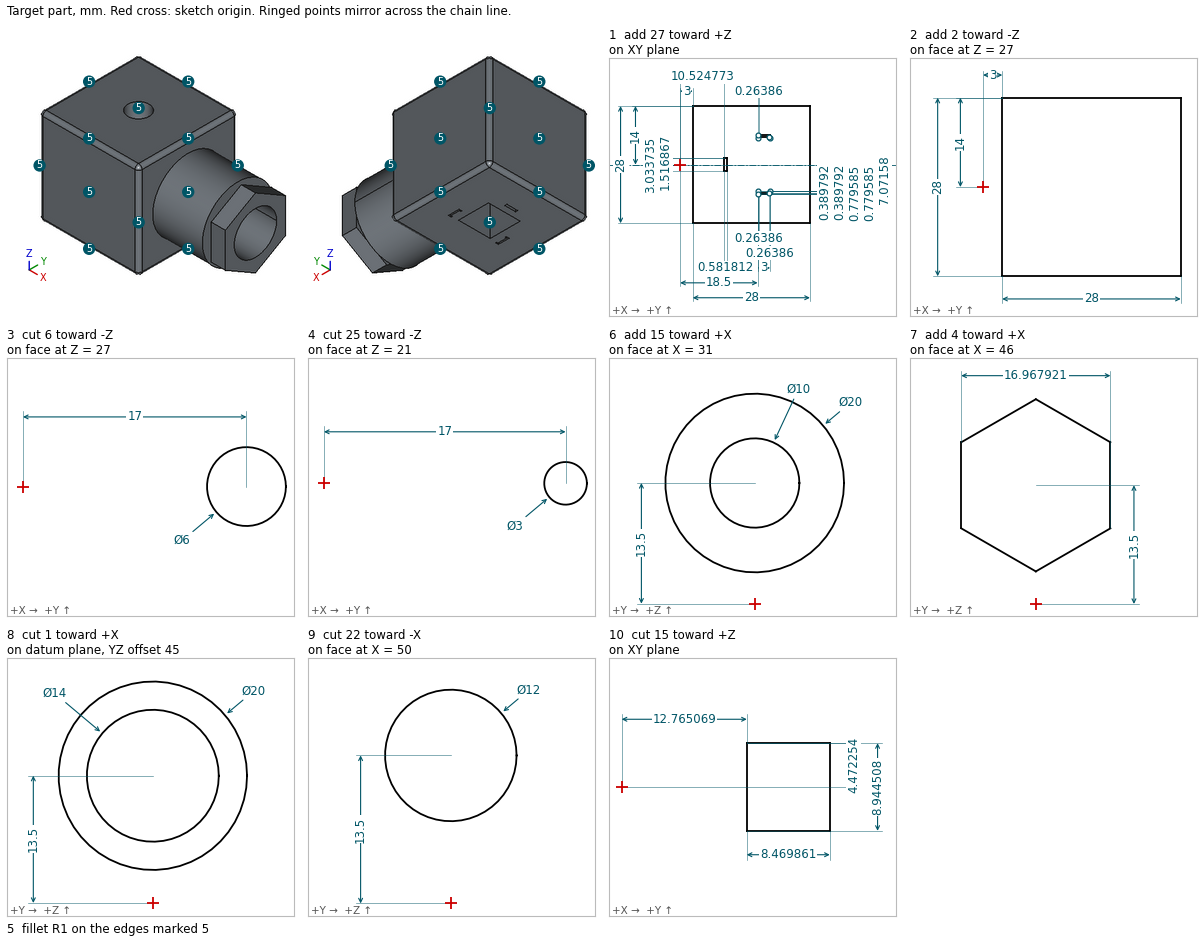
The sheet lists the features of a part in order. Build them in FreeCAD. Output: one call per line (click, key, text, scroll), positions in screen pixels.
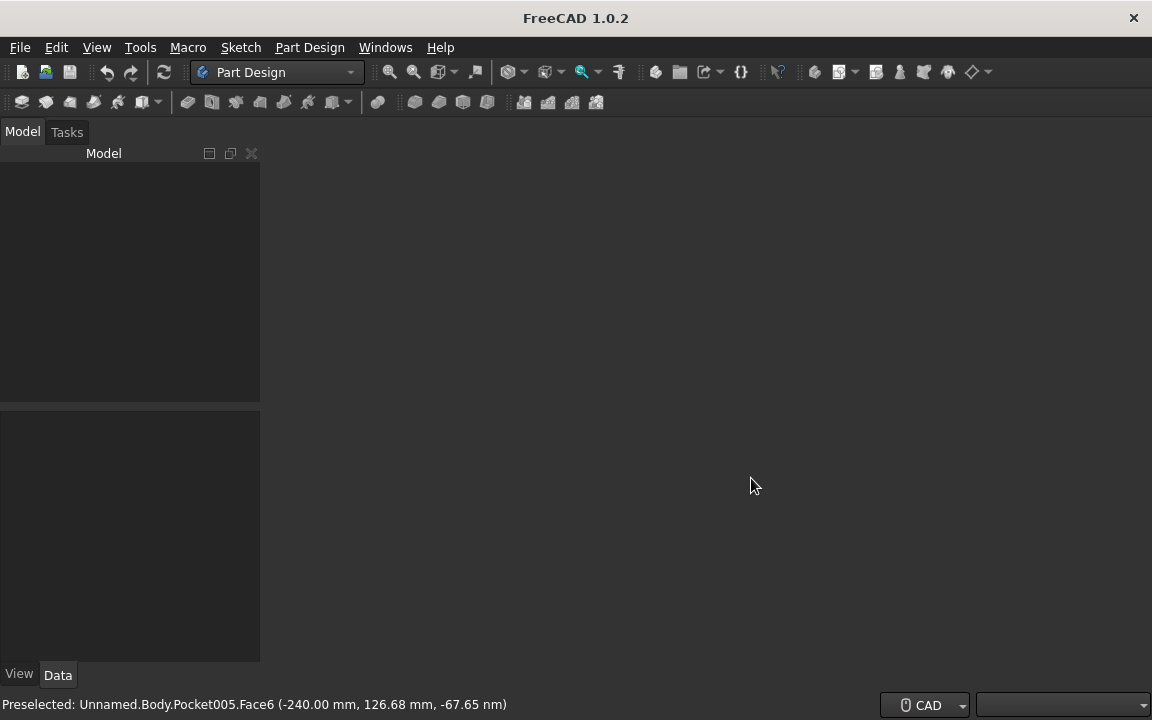
click(22, 72)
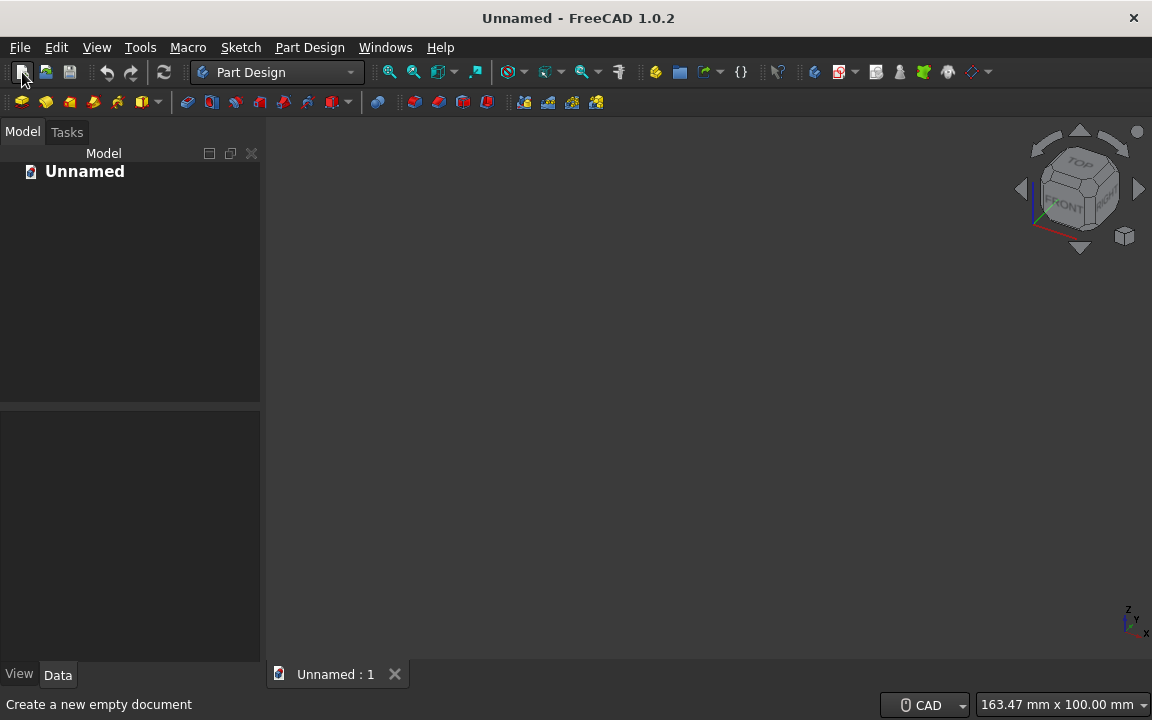
click(840, 72)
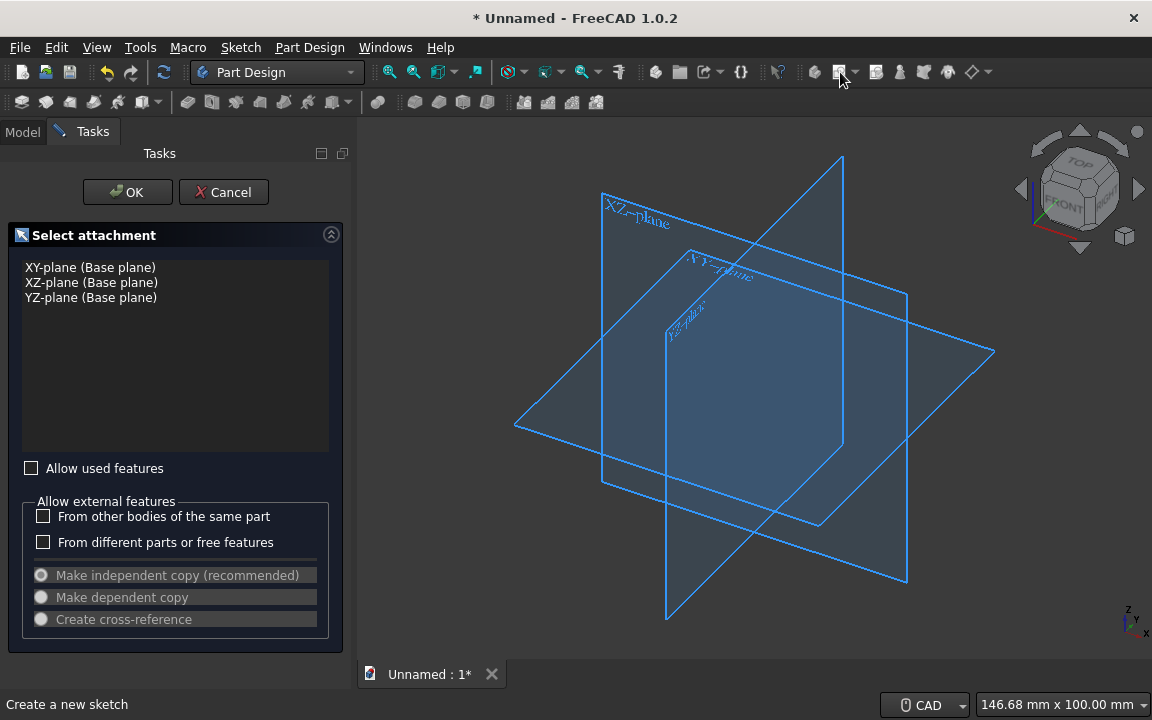
click(82, 268)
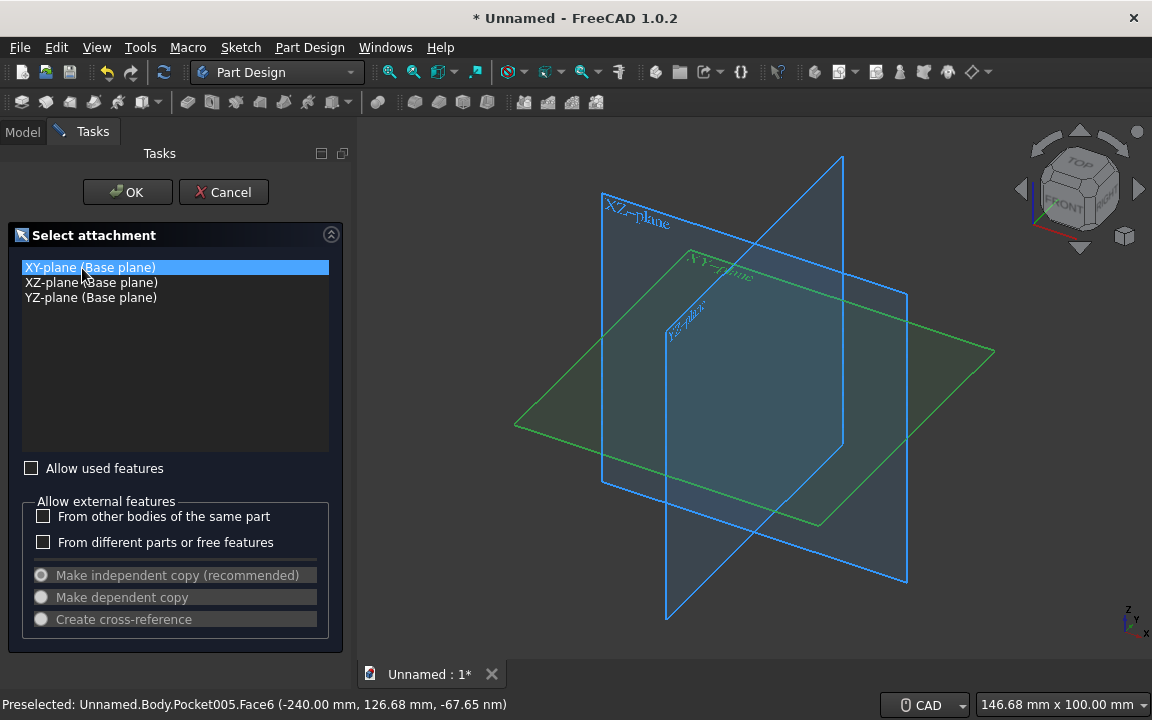
click(128, 192)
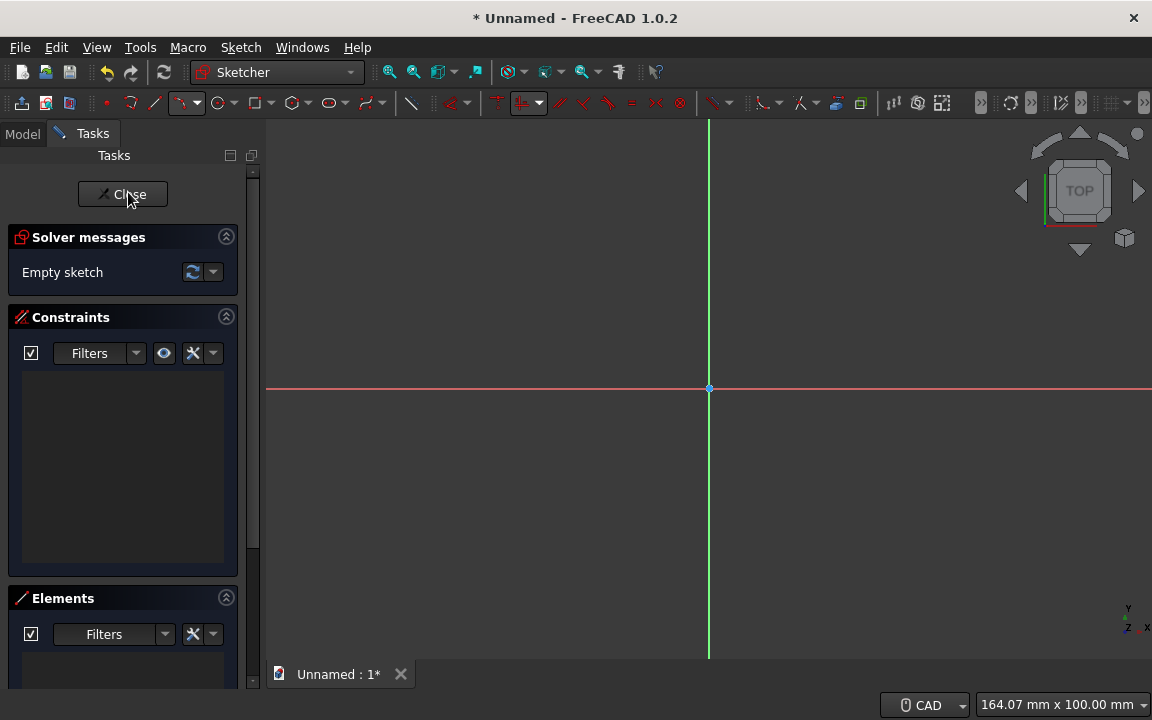
scroll(917, 389, up, 4)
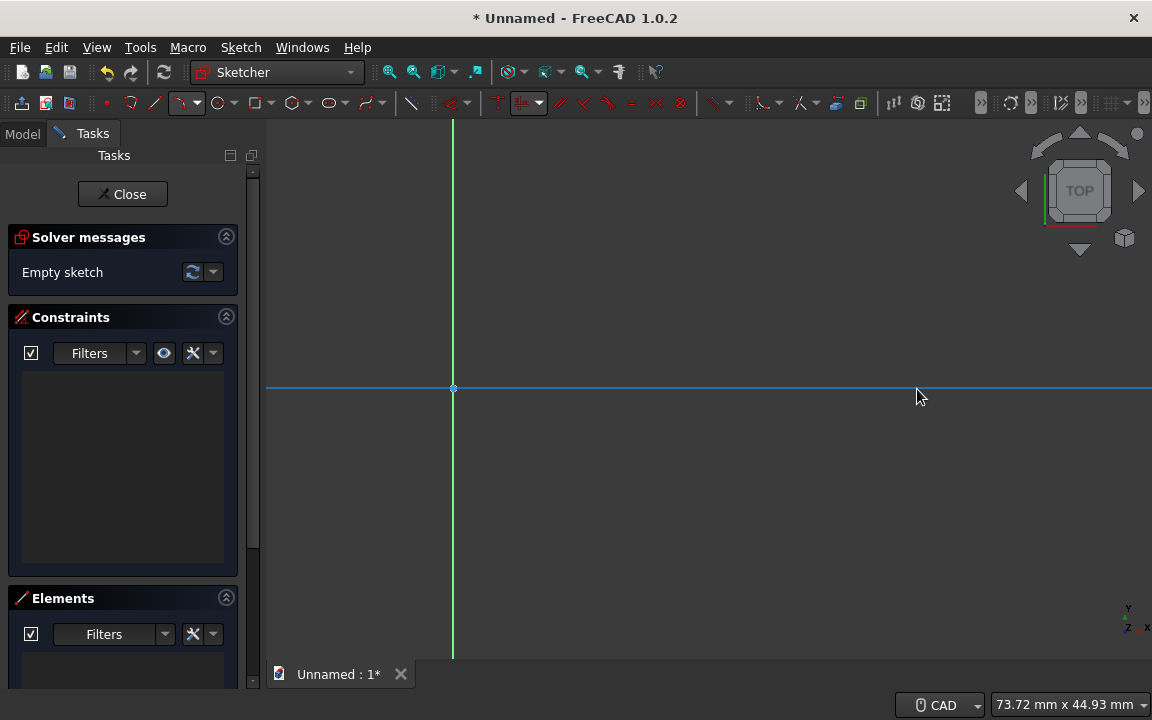
click(256, 104)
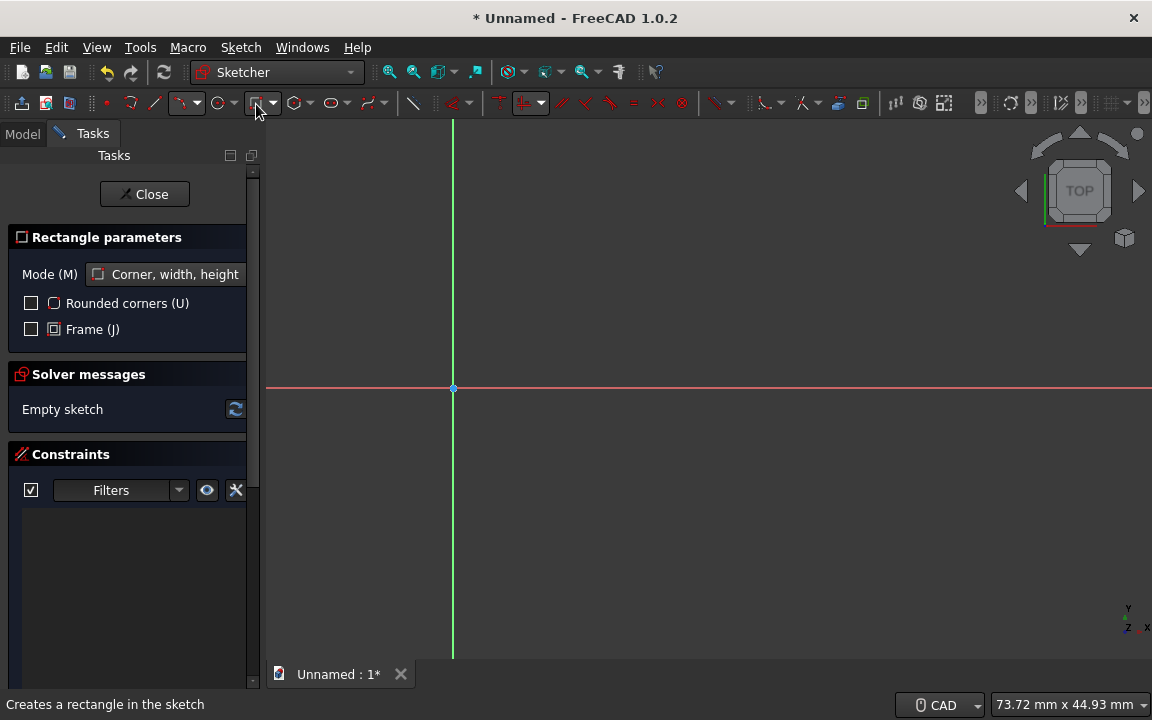
click(489, 220)
click(826, 557)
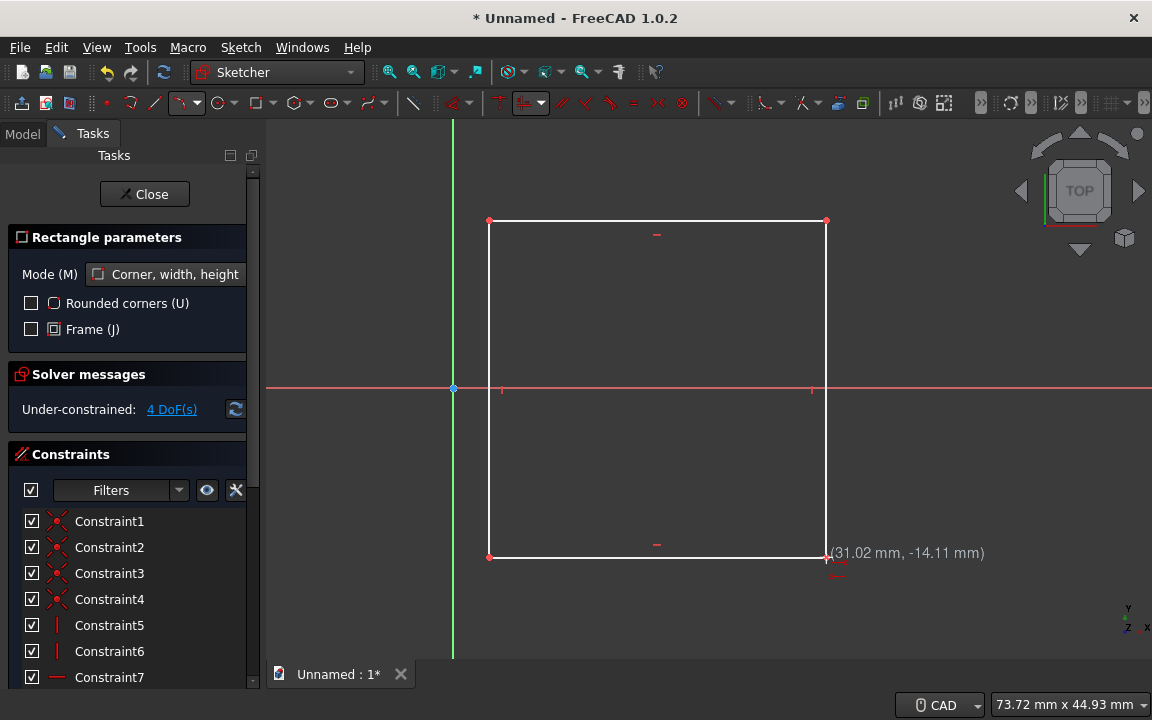
click(132, 104)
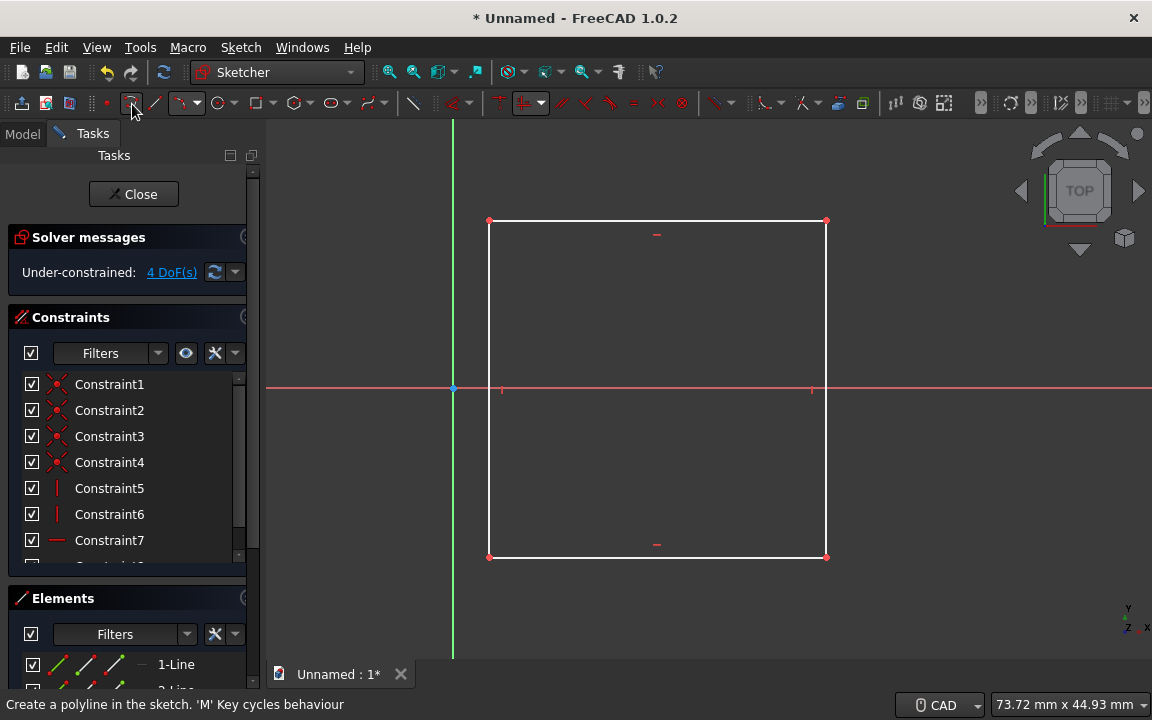
click(676, 464)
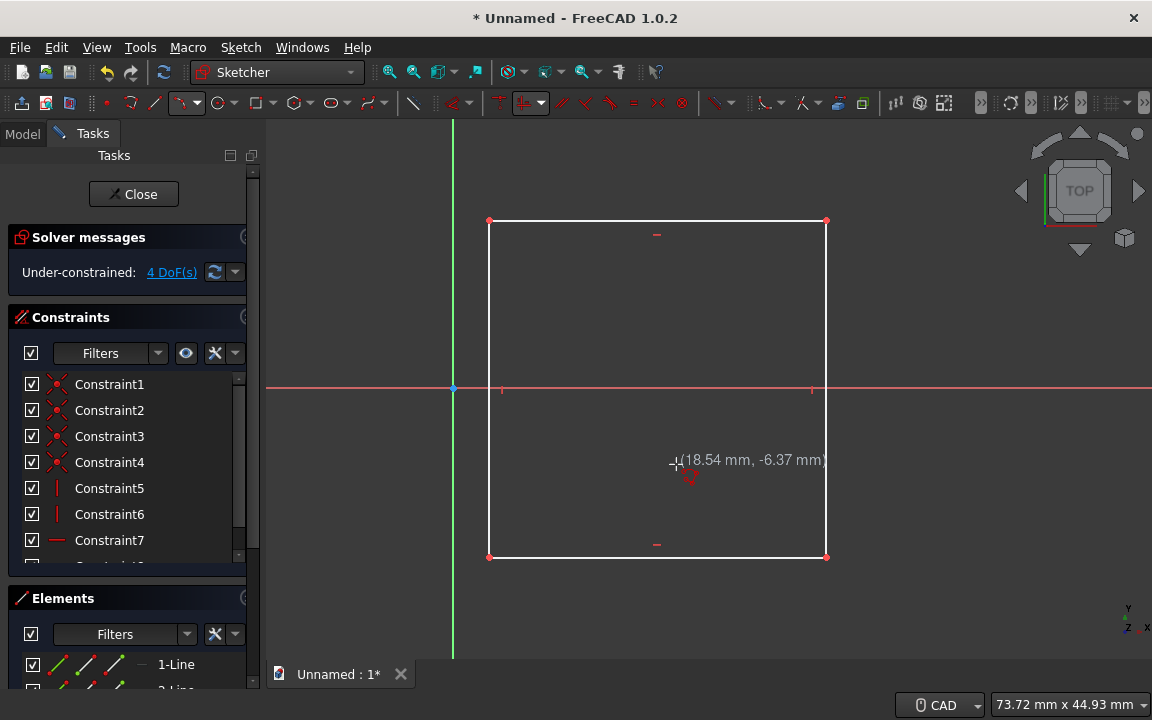
scroll(679, 464, up, 9)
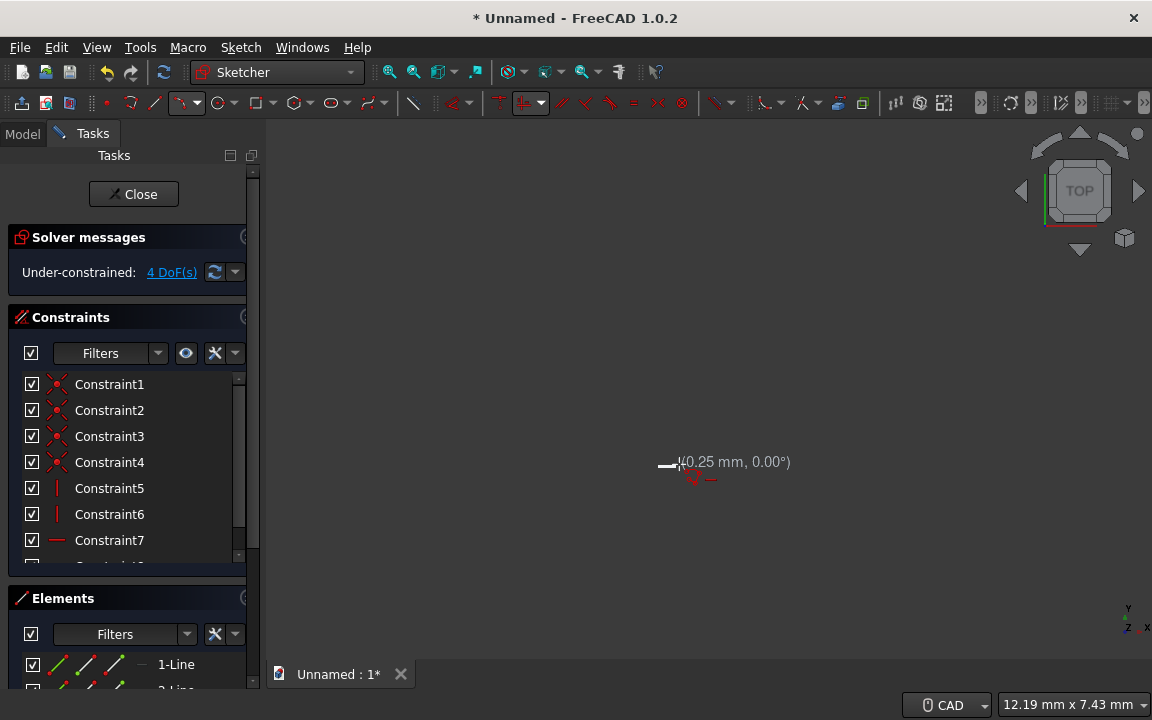
click(675, 461)
click(675, 489)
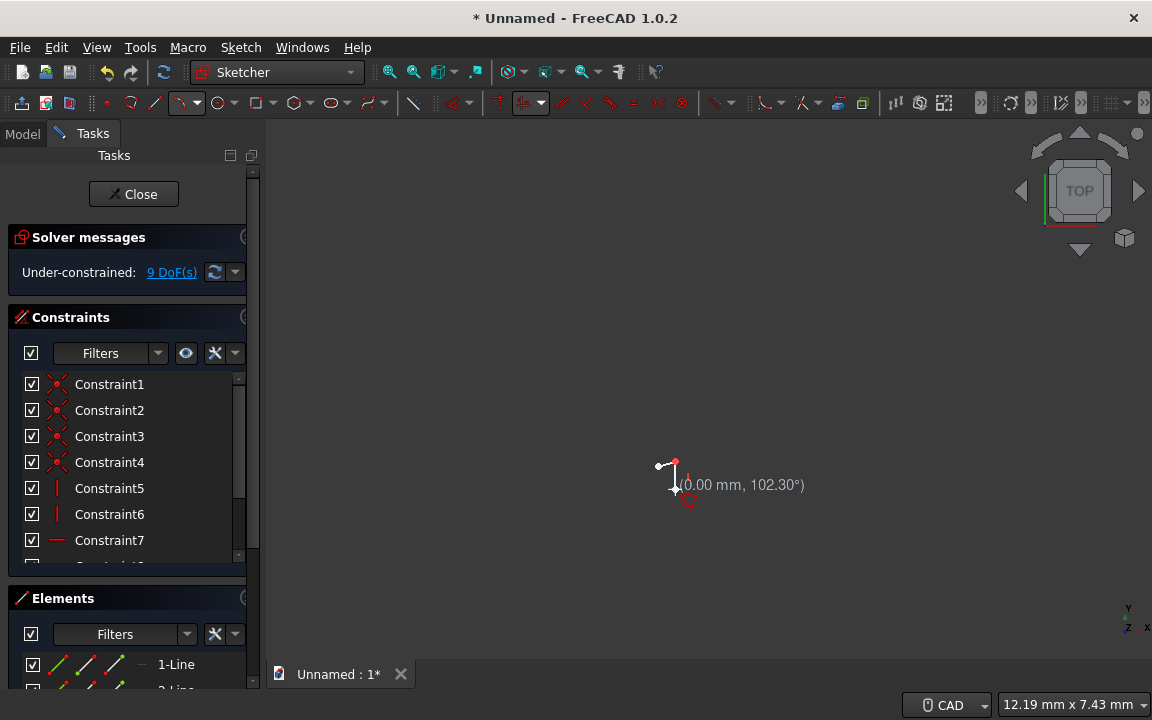
scroll(681, 465, down, 9)